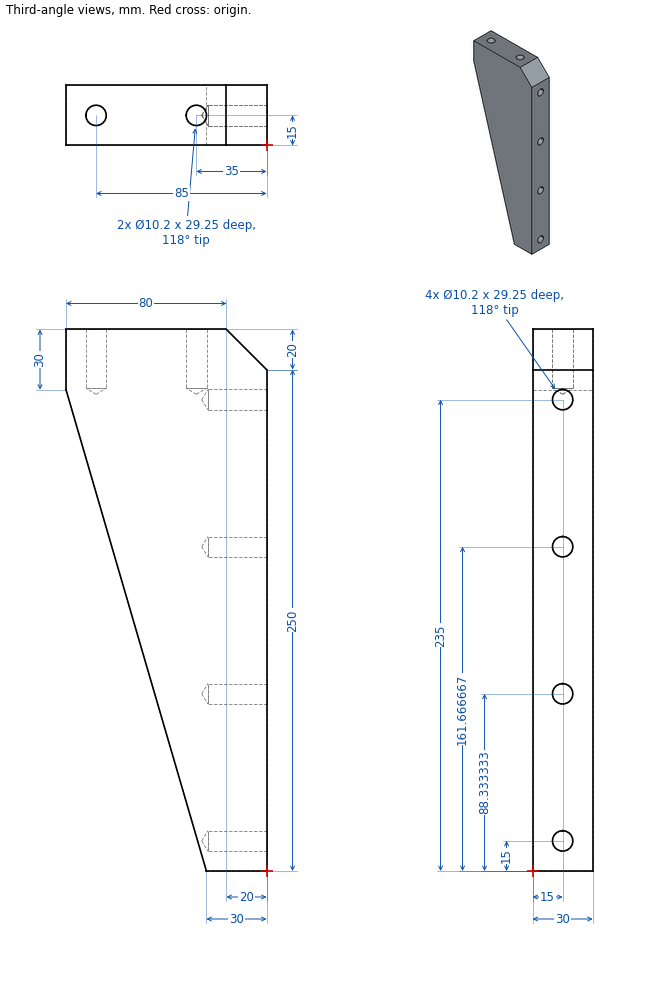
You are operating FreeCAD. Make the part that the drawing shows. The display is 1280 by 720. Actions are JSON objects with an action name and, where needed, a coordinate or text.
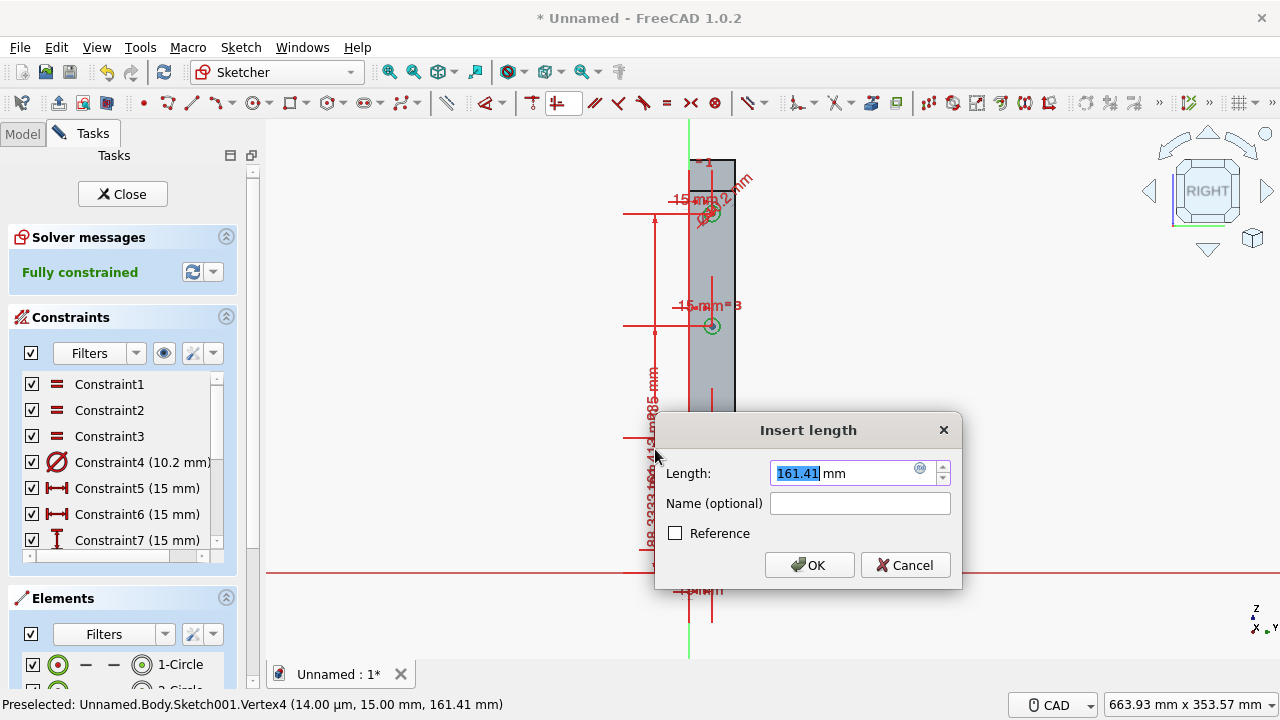
{"action": "type", "text": "161.666667"}
{"action": "key", "text": "Return"}
{"action": "key", "text": "Escape"}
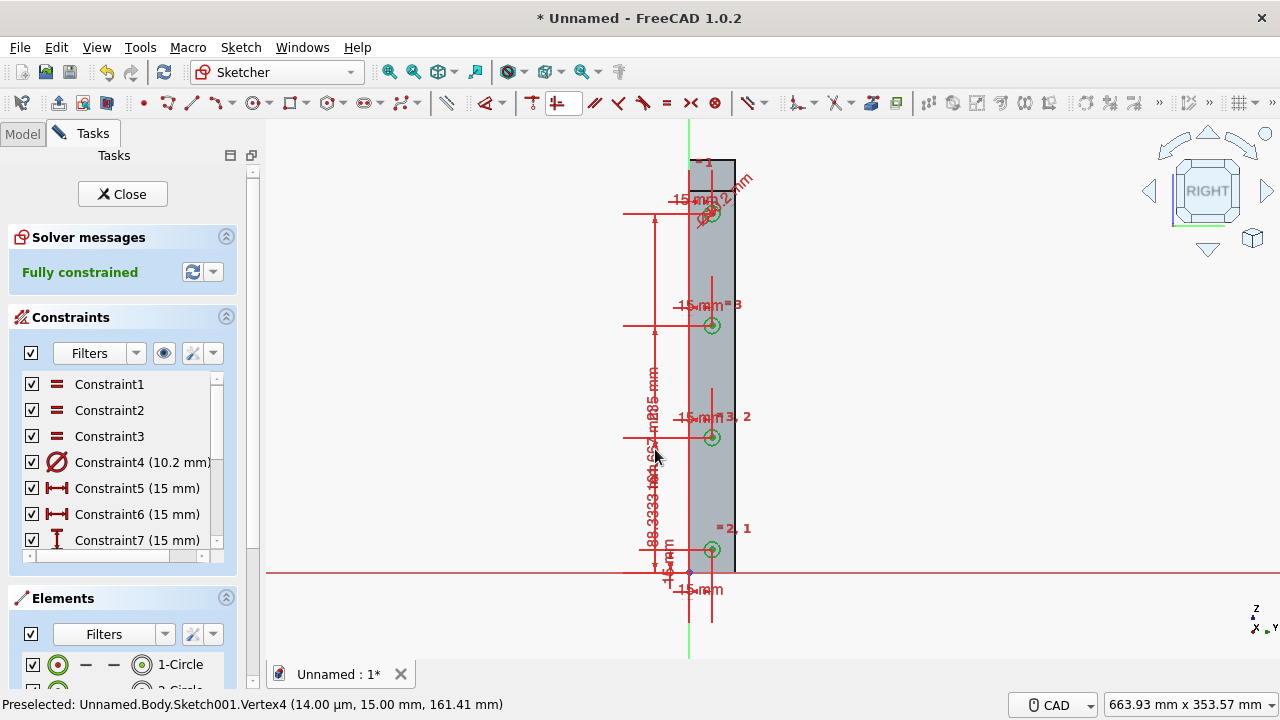
{"action": "left_click", "coordinate": [123, 194]}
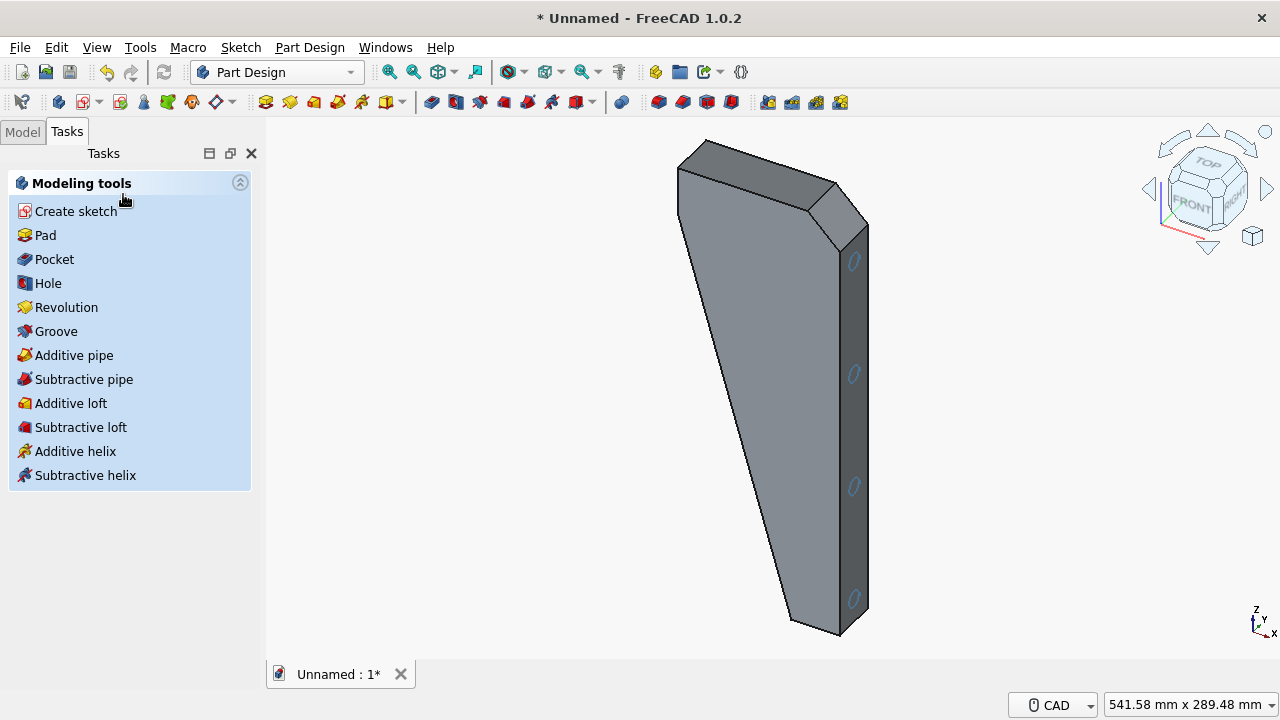
{"action": "left_click", "coordinate": [456, 102]}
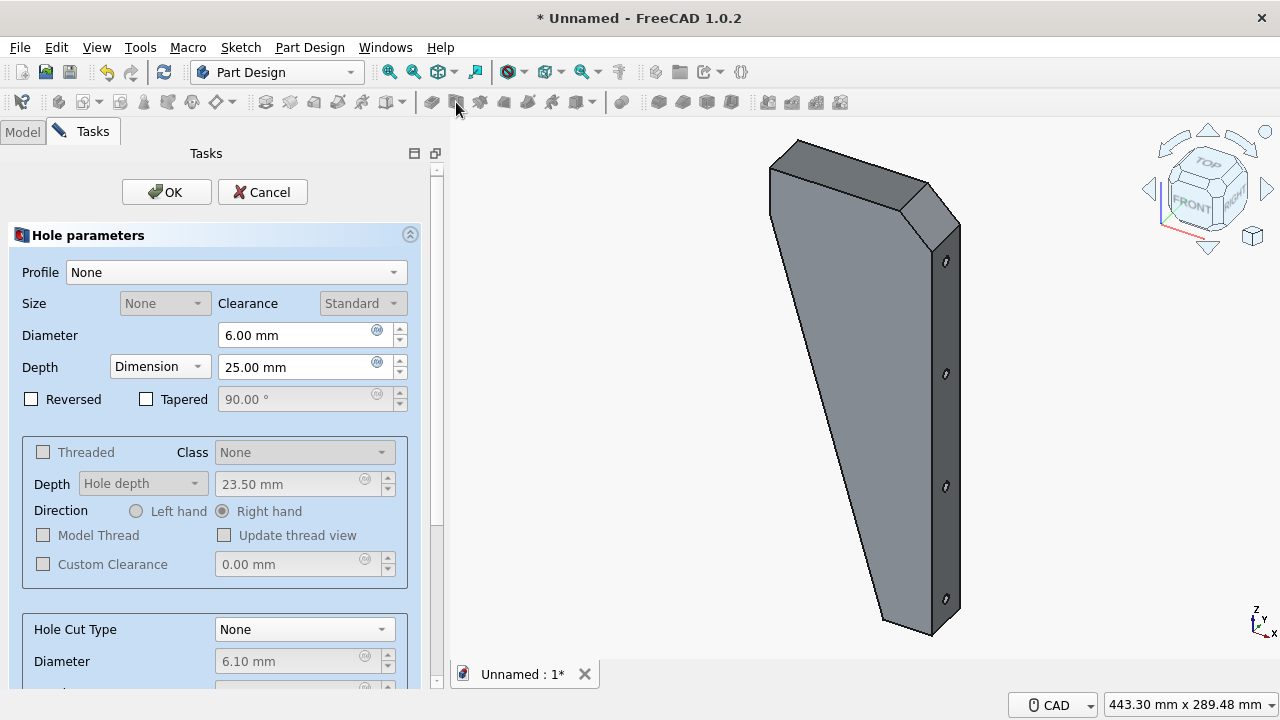
{"action": "triple_click", "coordinate": [305, 335]}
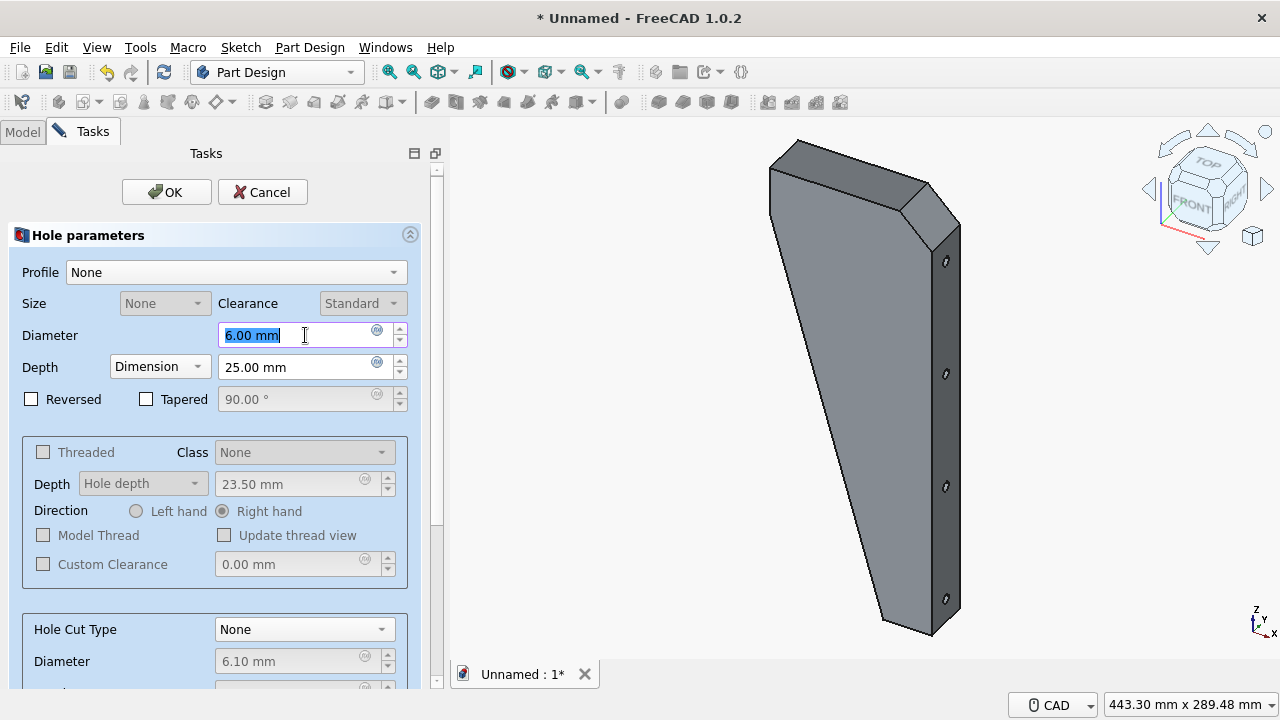
{"action": "type", "text": "10.2"}
{"action": "key", "text": "Tab"}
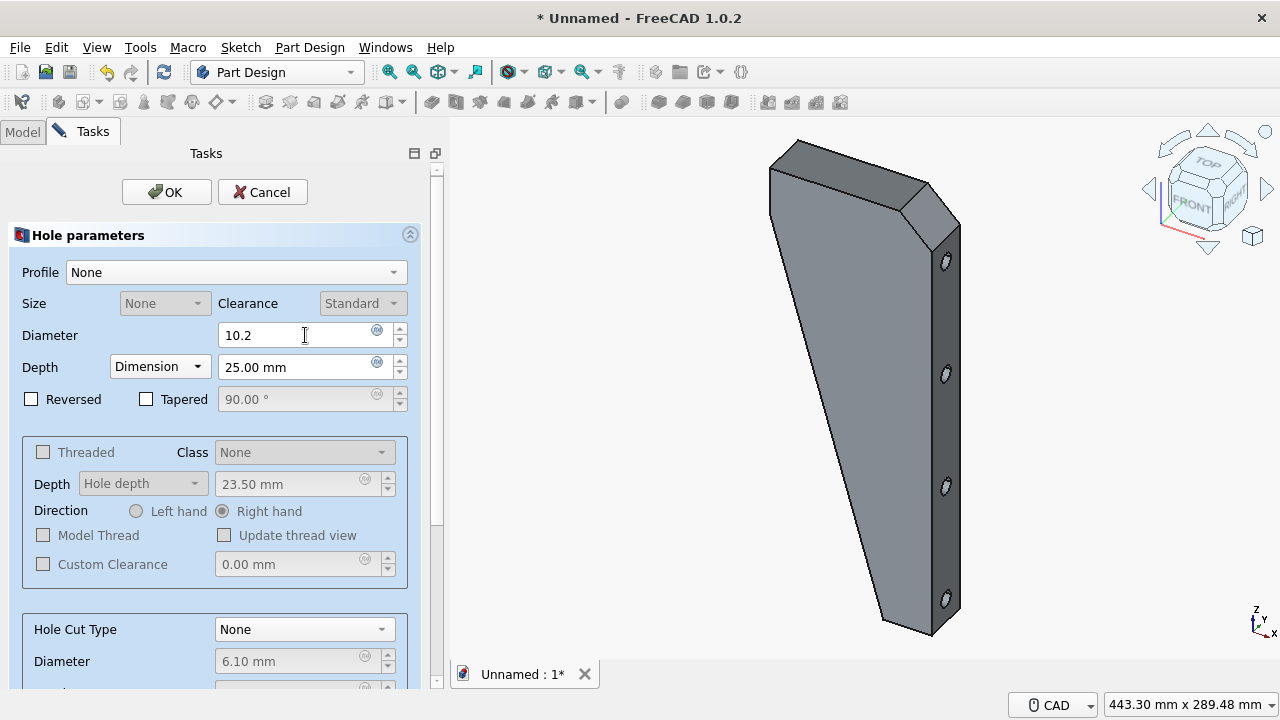
{"action": "triple_click", "coordinate": [305, 367]}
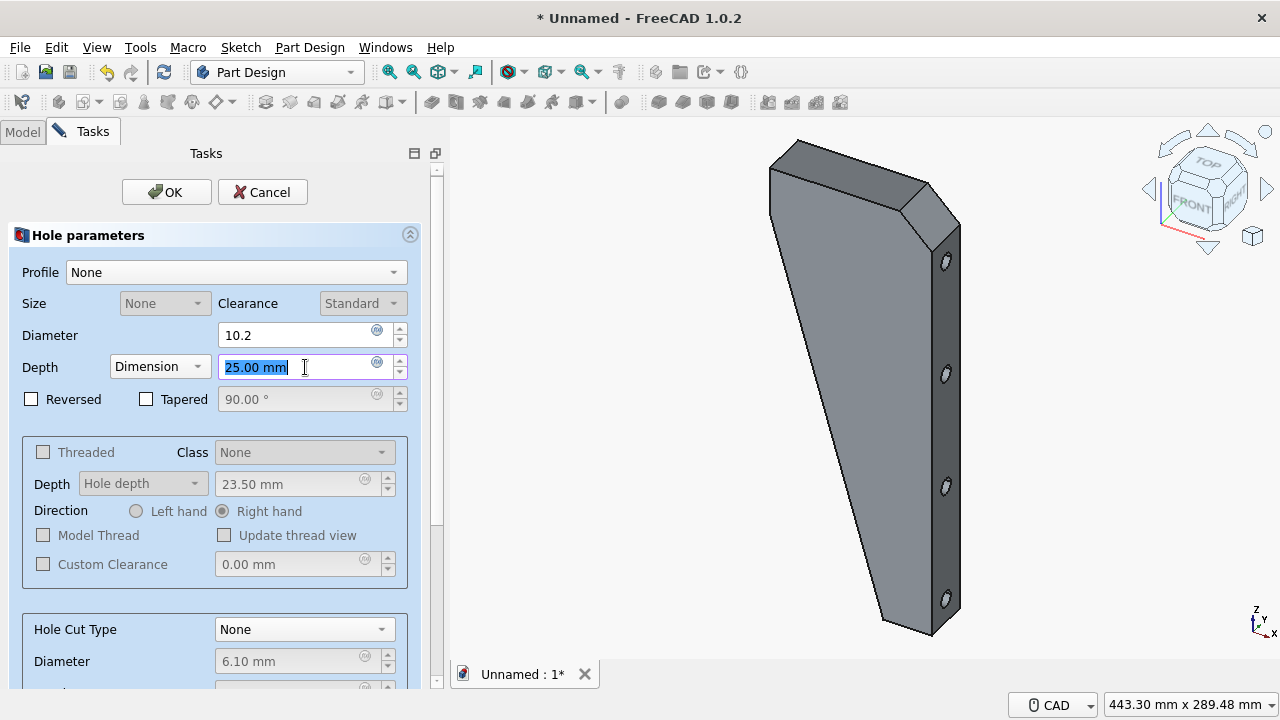
{"action": "type", "text": "29.25"}
{"action": "key", "text": "Tab"}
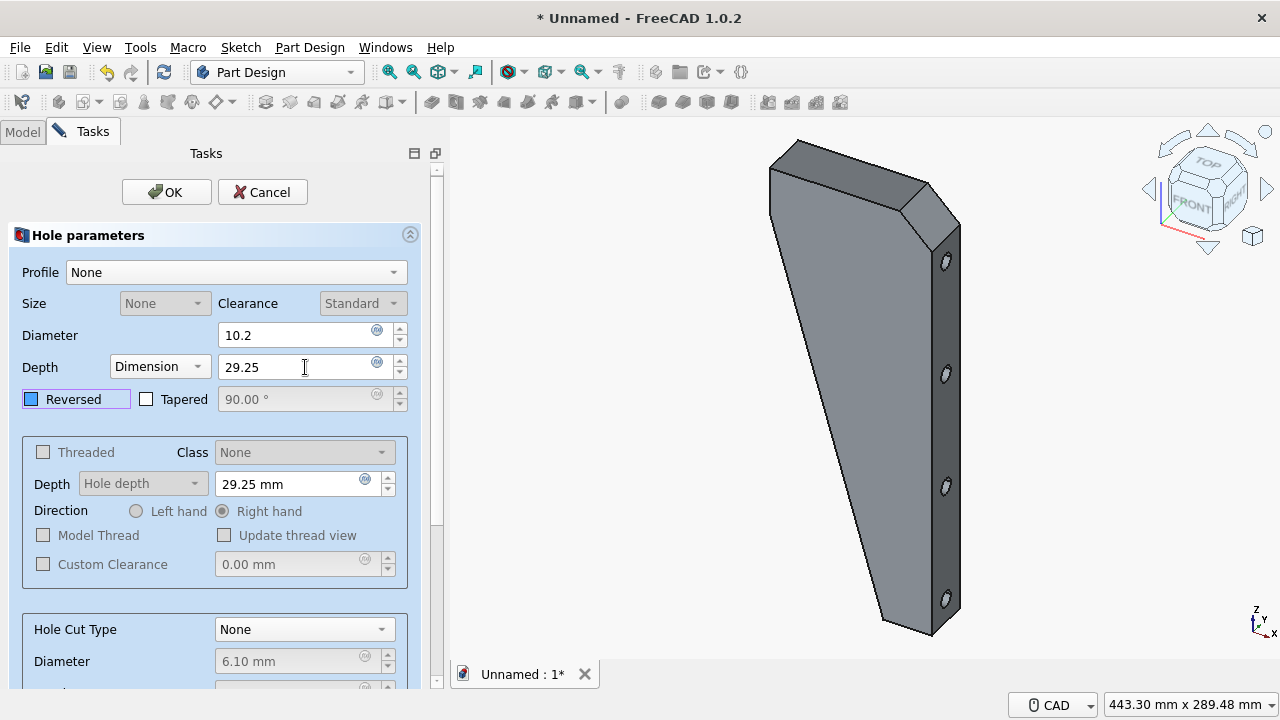
{"action": "left_click", "coordinate": [167, 192]}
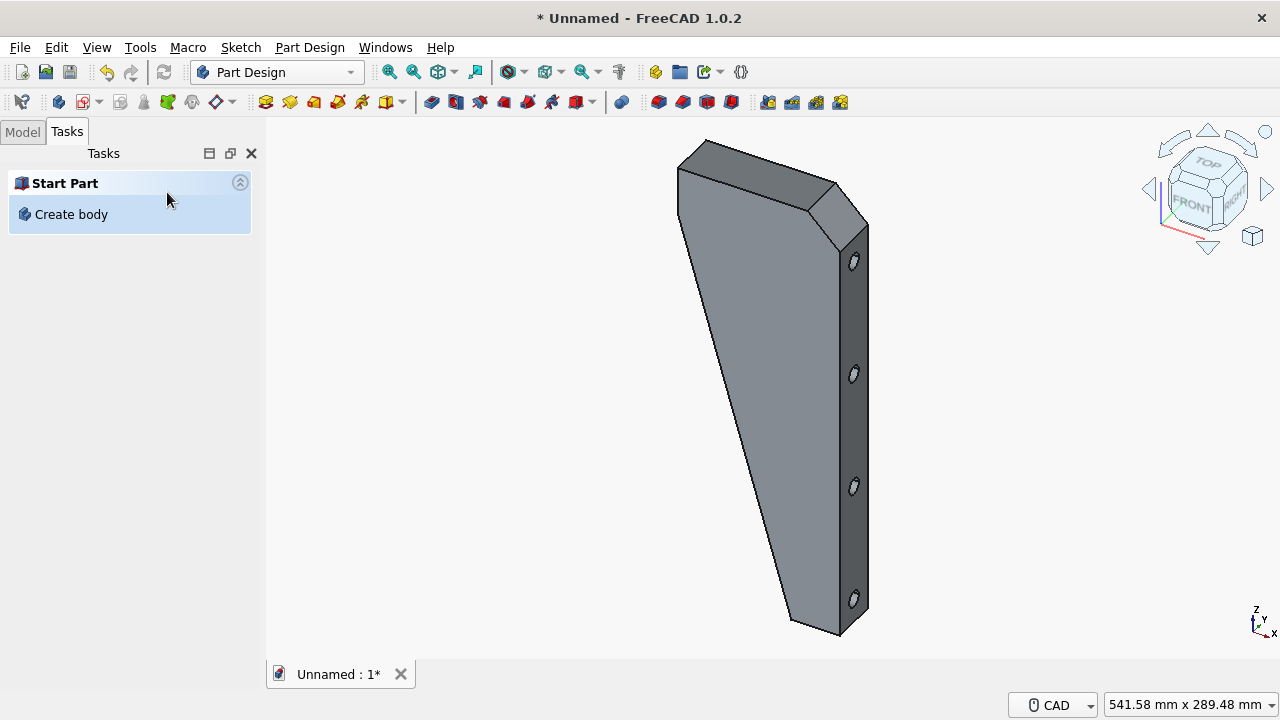
{"action": "left_click", "coordinate": [794, 187]}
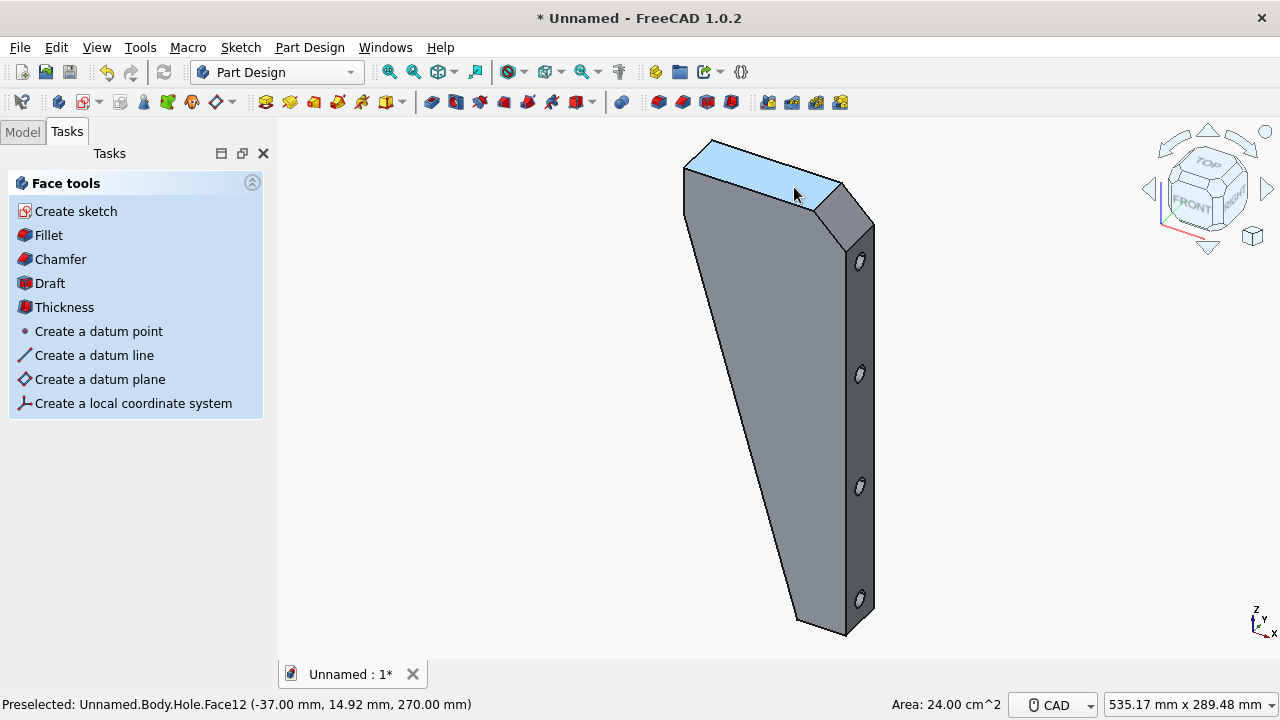
{"action": "left_click", "coordinate": [84, 102]}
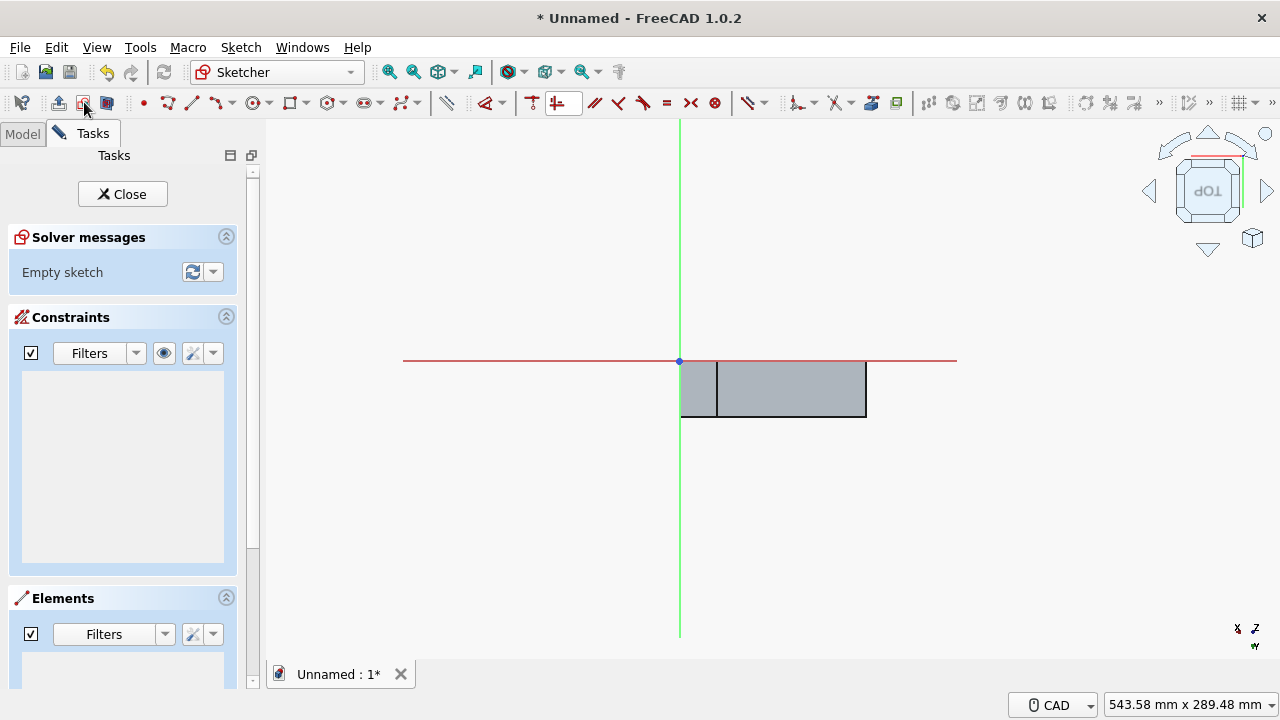
{"action": "scroll", "coordinate": [789, 376], "scroll_direction": "up", "scroll_amount": 6}